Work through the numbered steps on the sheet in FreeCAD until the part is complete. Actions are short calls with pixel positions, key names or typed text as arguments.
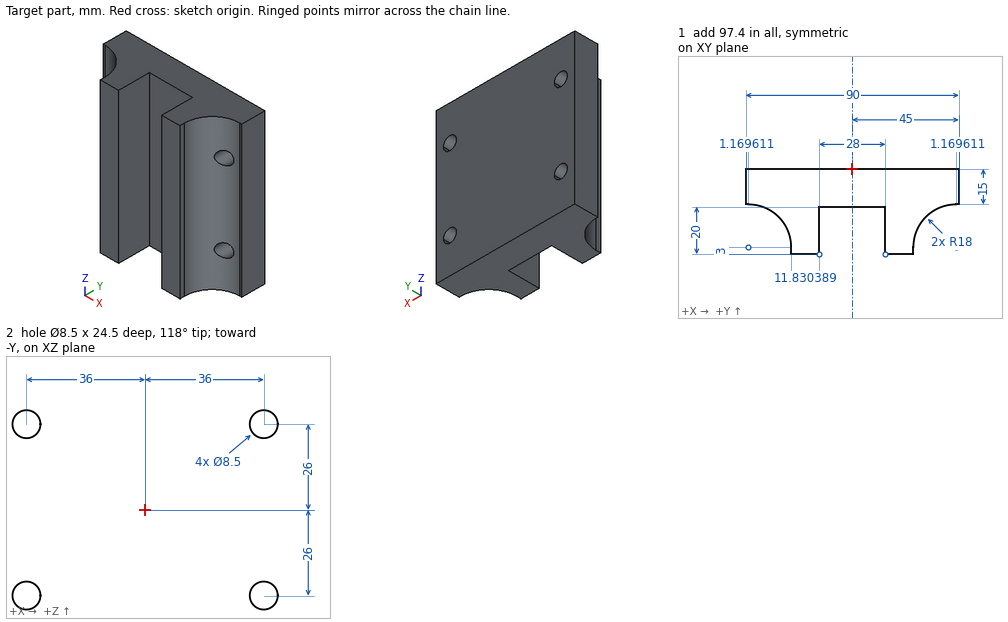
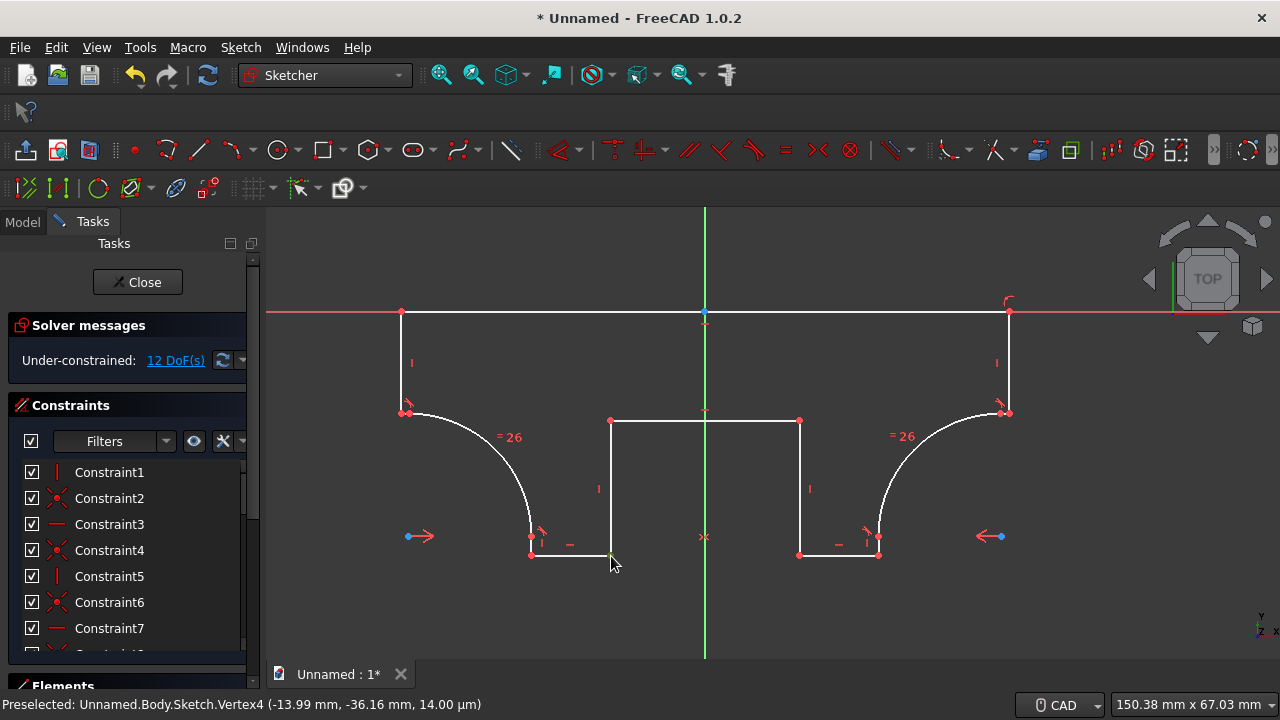
click(800, 556)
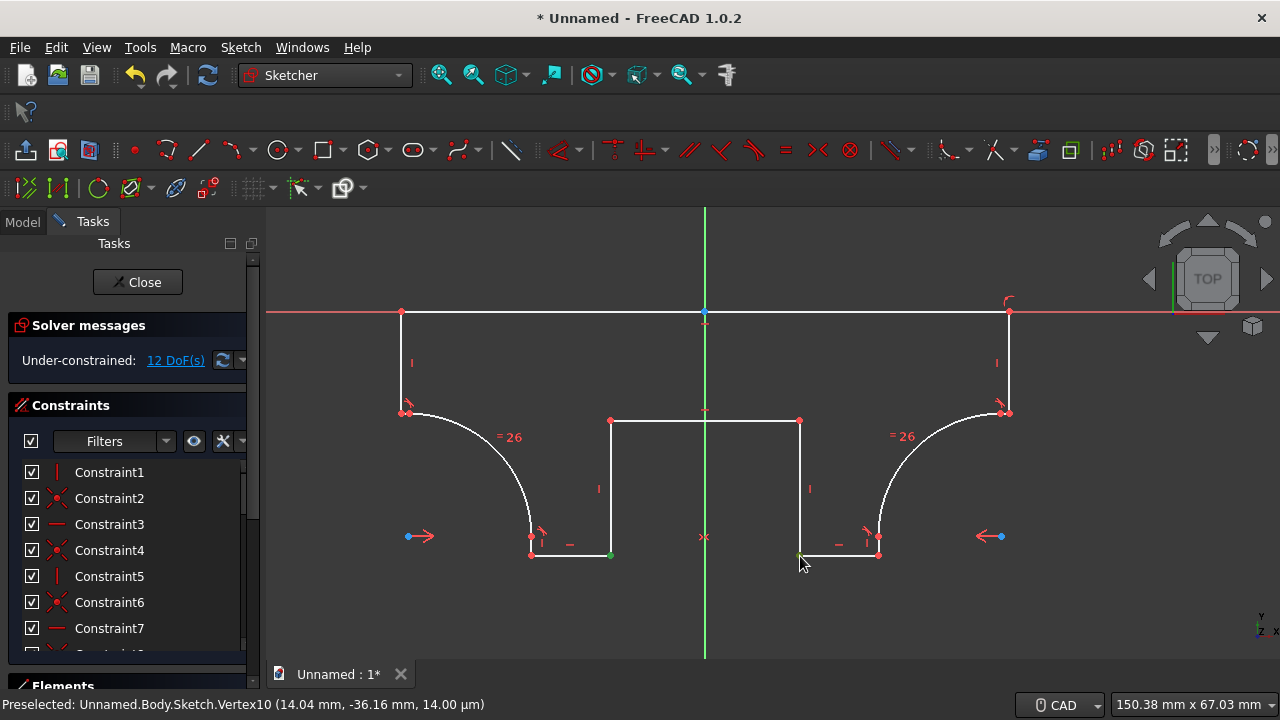
click(705, 603)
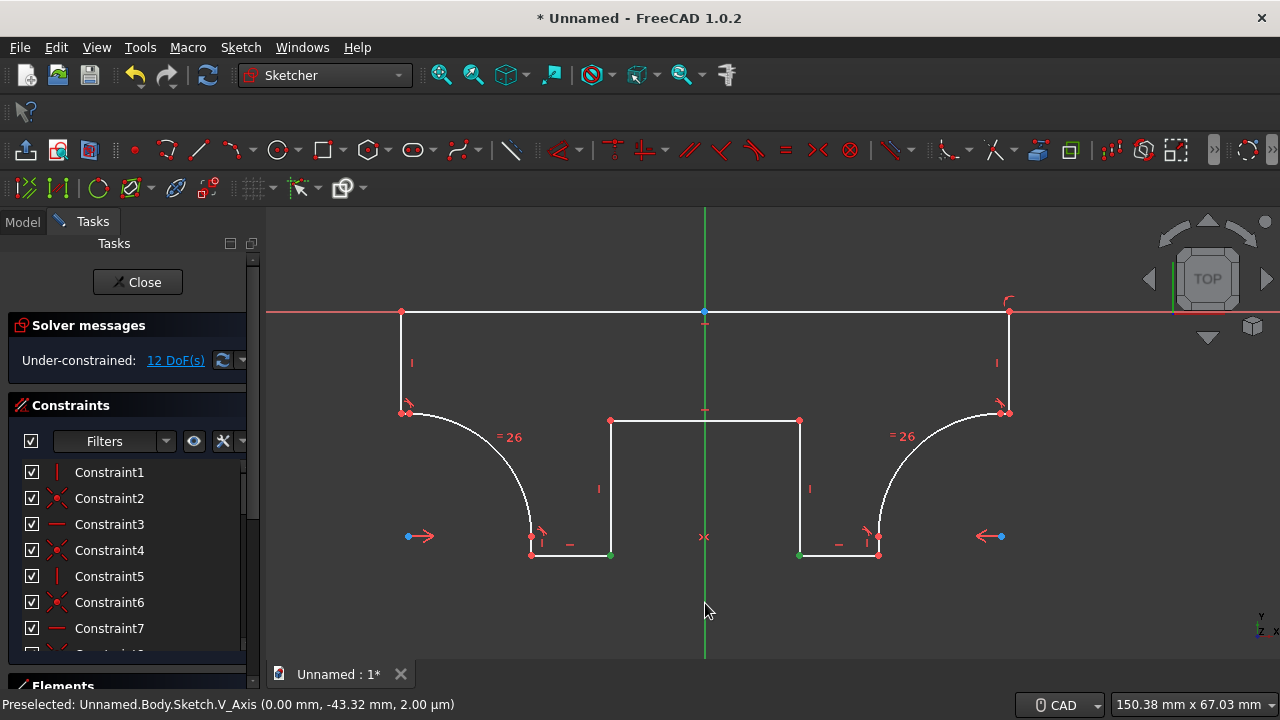
click(818, 150)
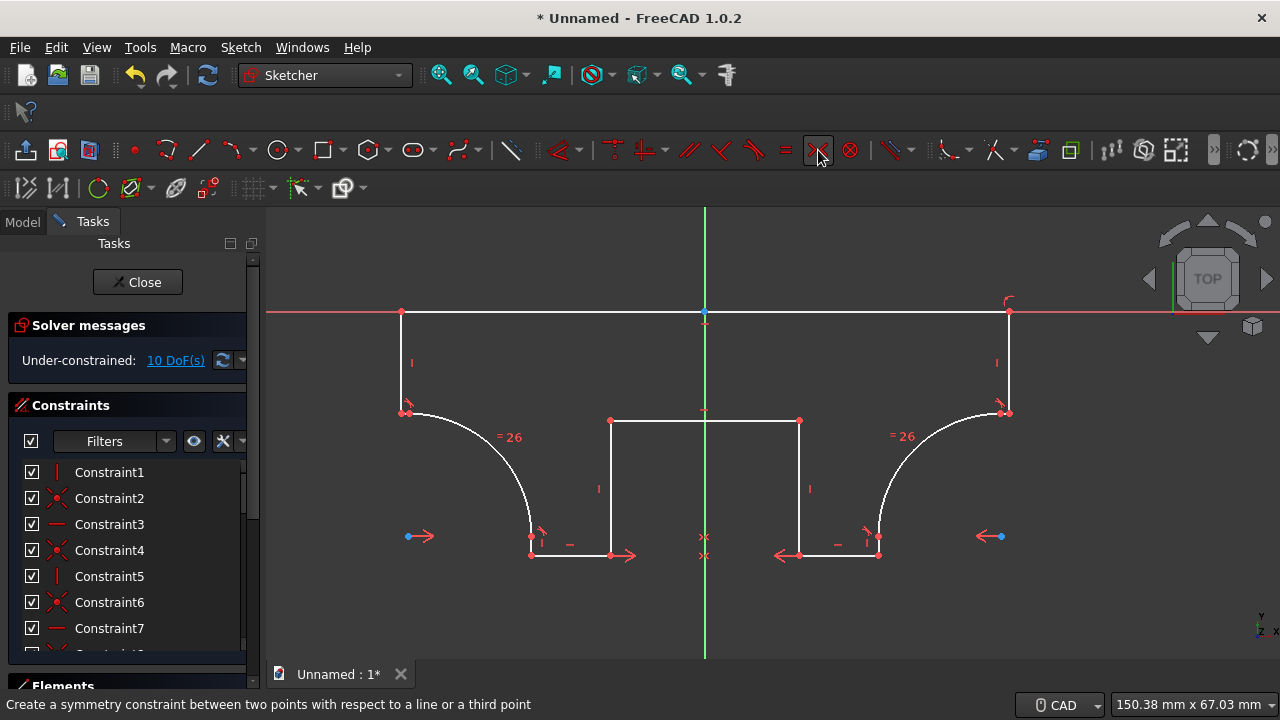
click(945, 427)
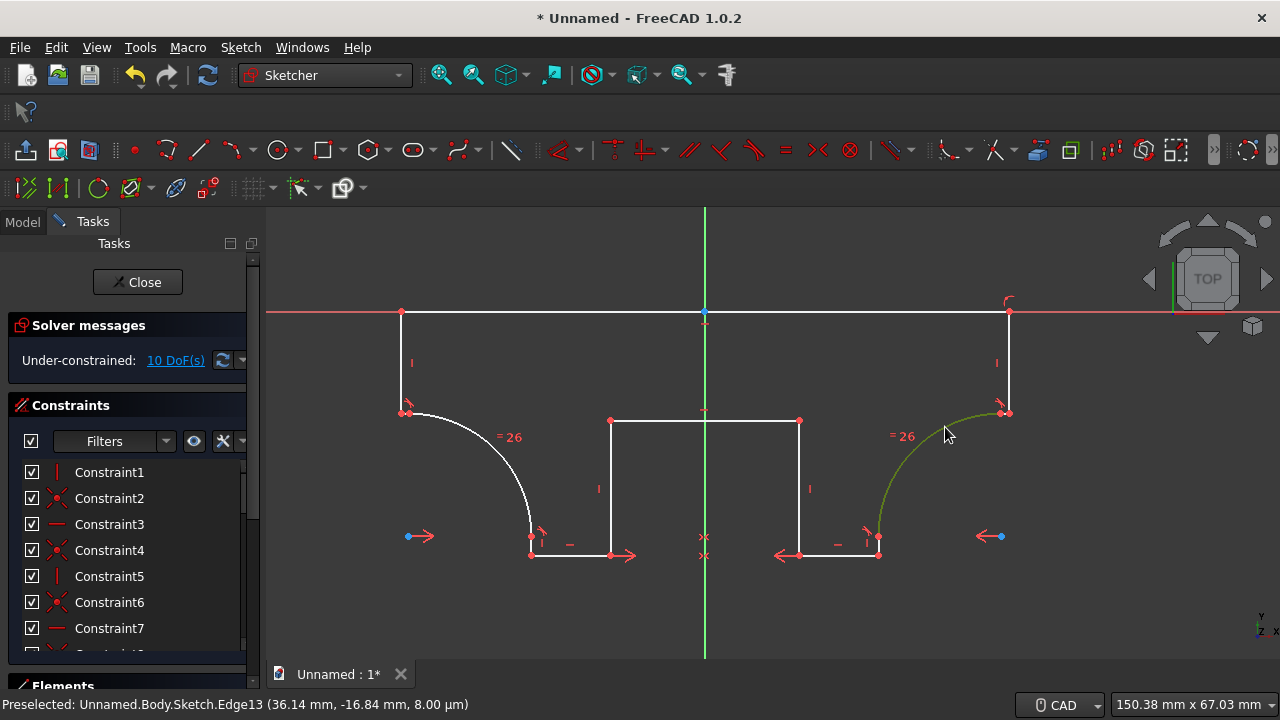
click(582, 150)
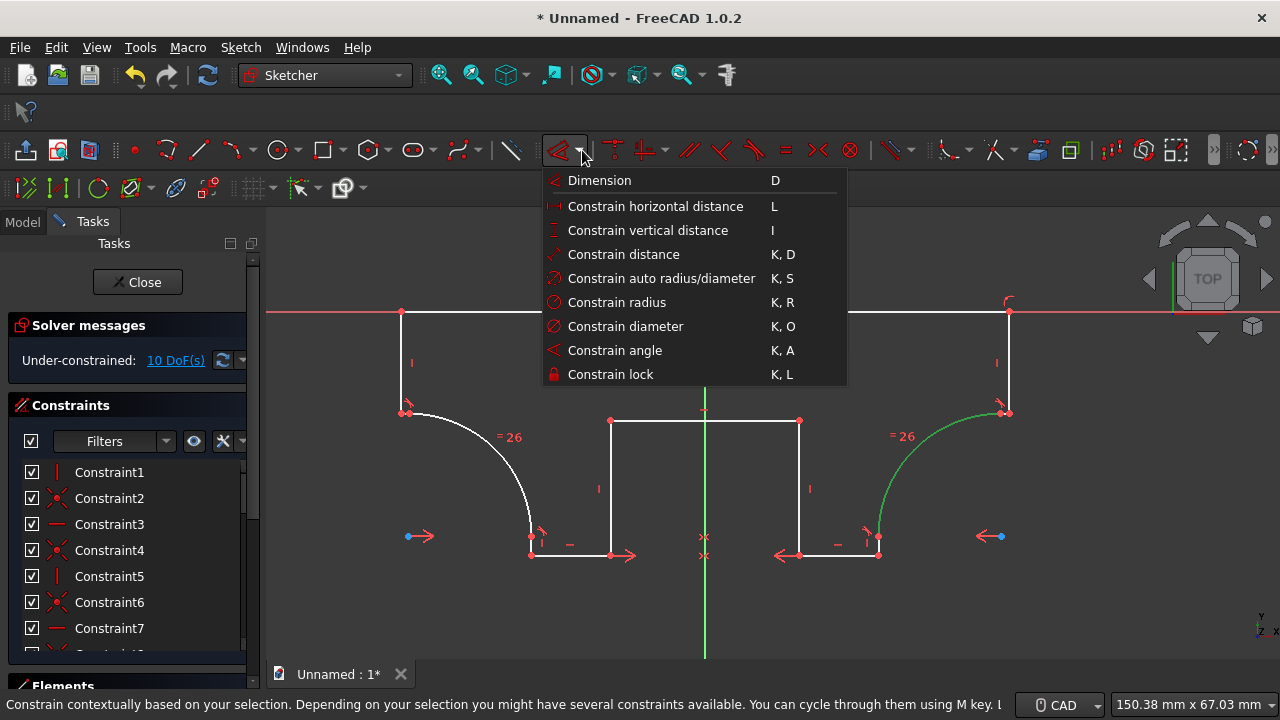
click(695, 302)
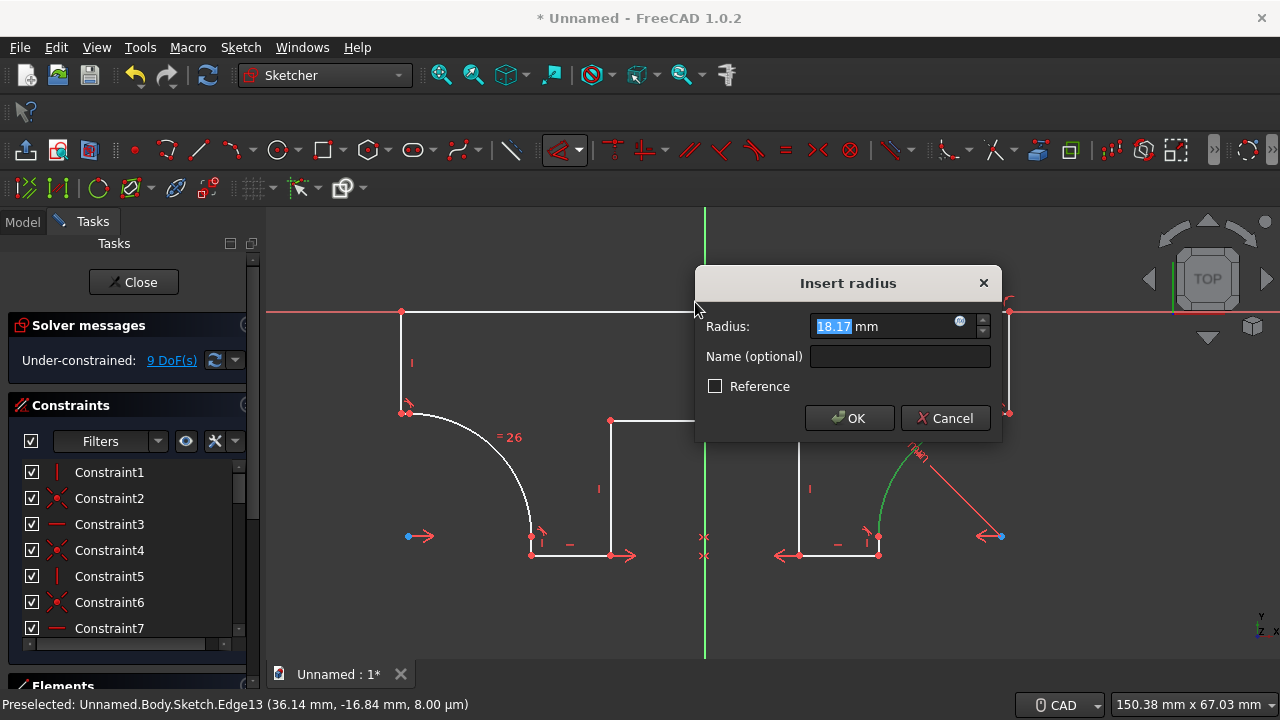
text(18)
key(Return)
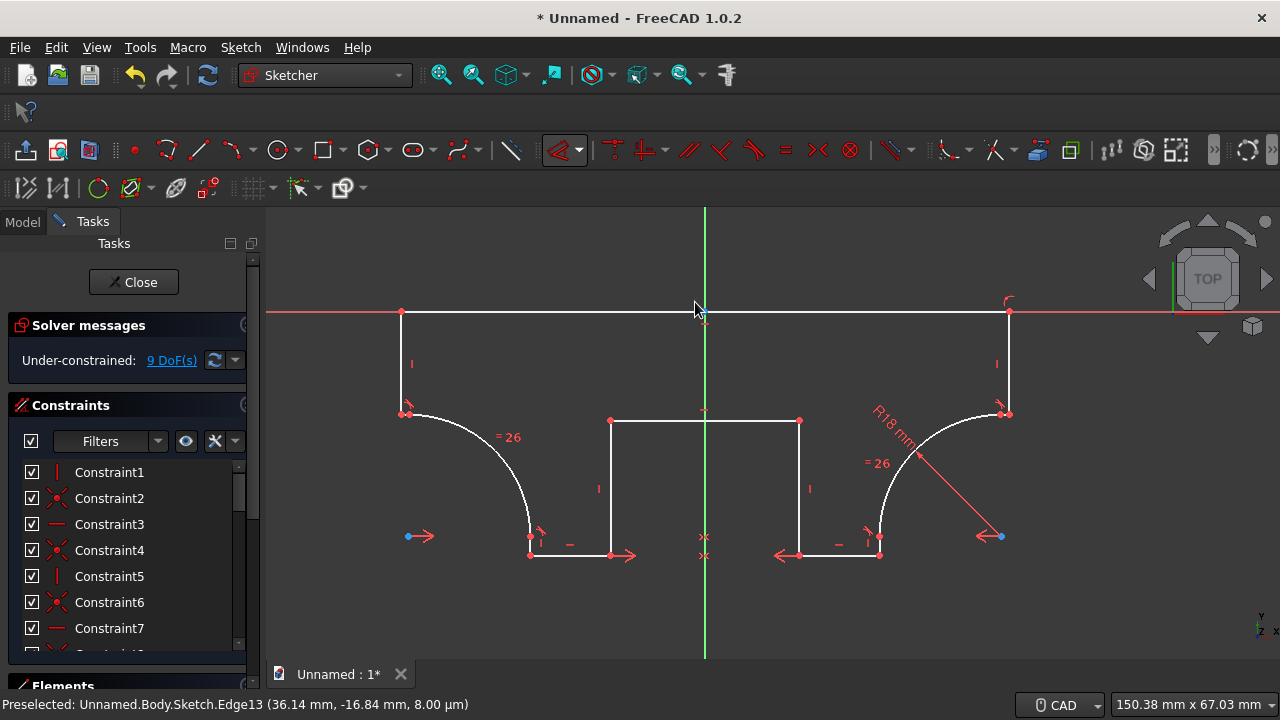
scroll(530, 546, up, 4)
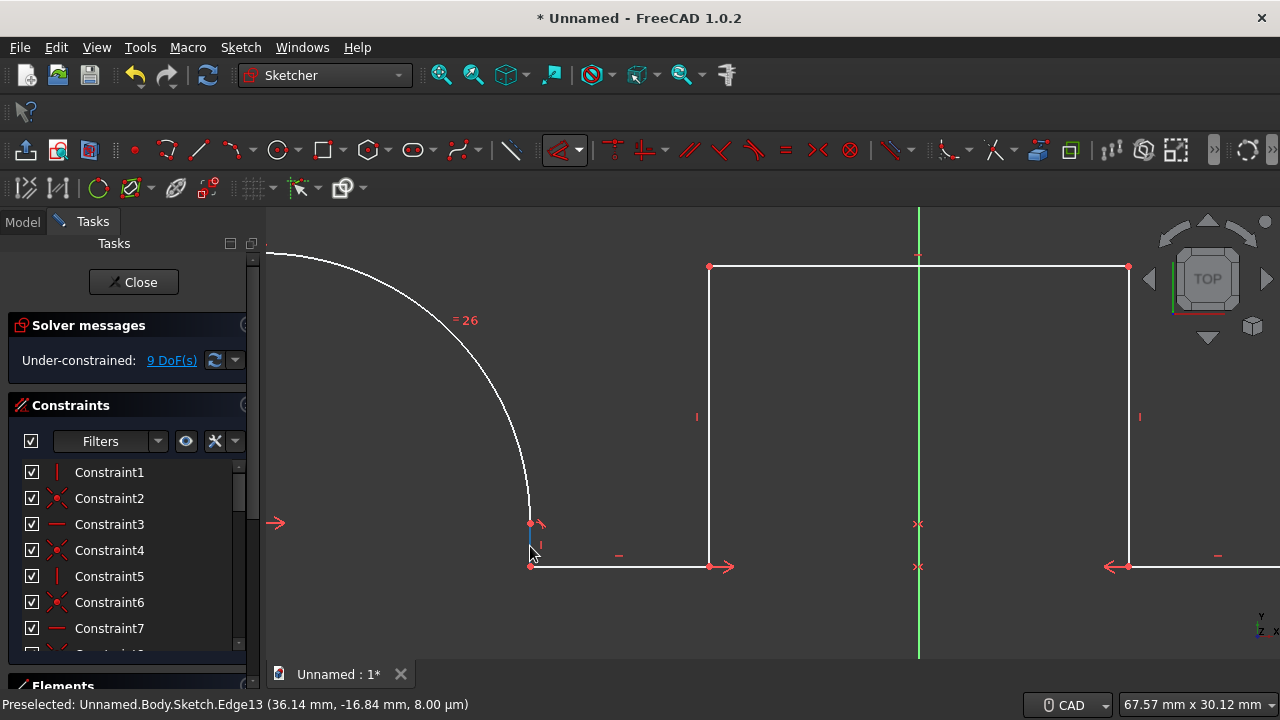
click(530, 545)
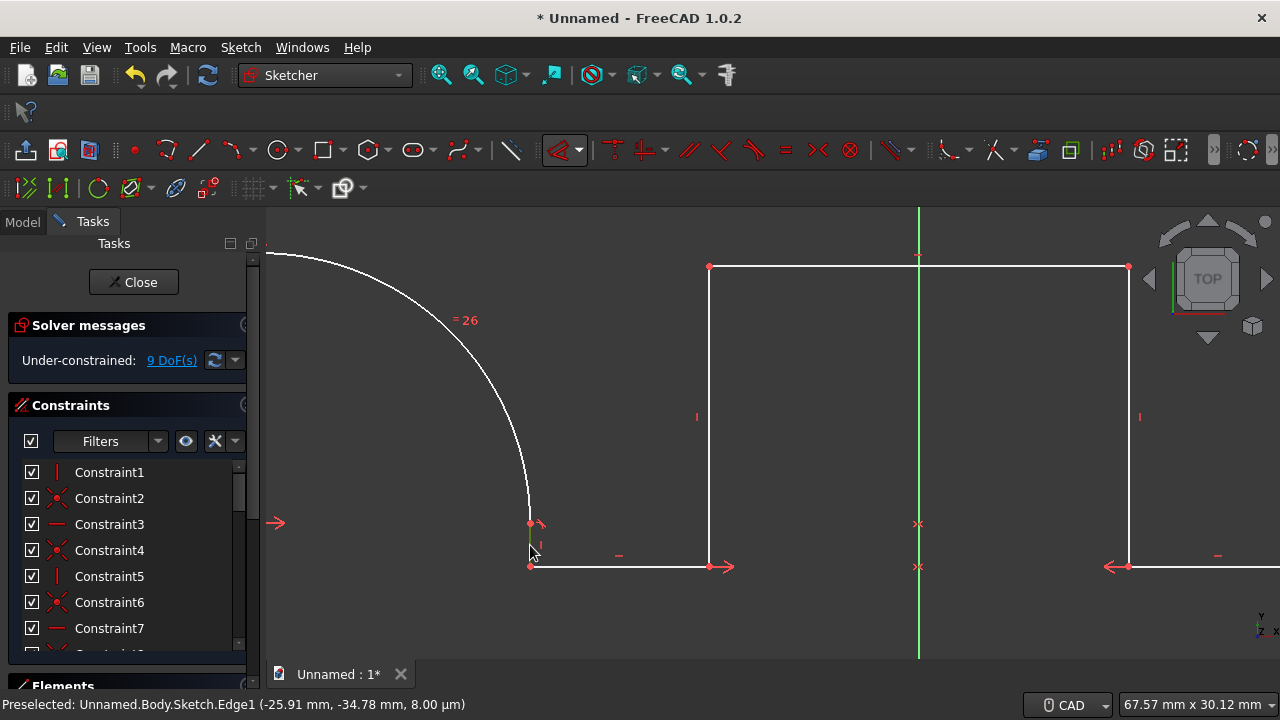
key(i)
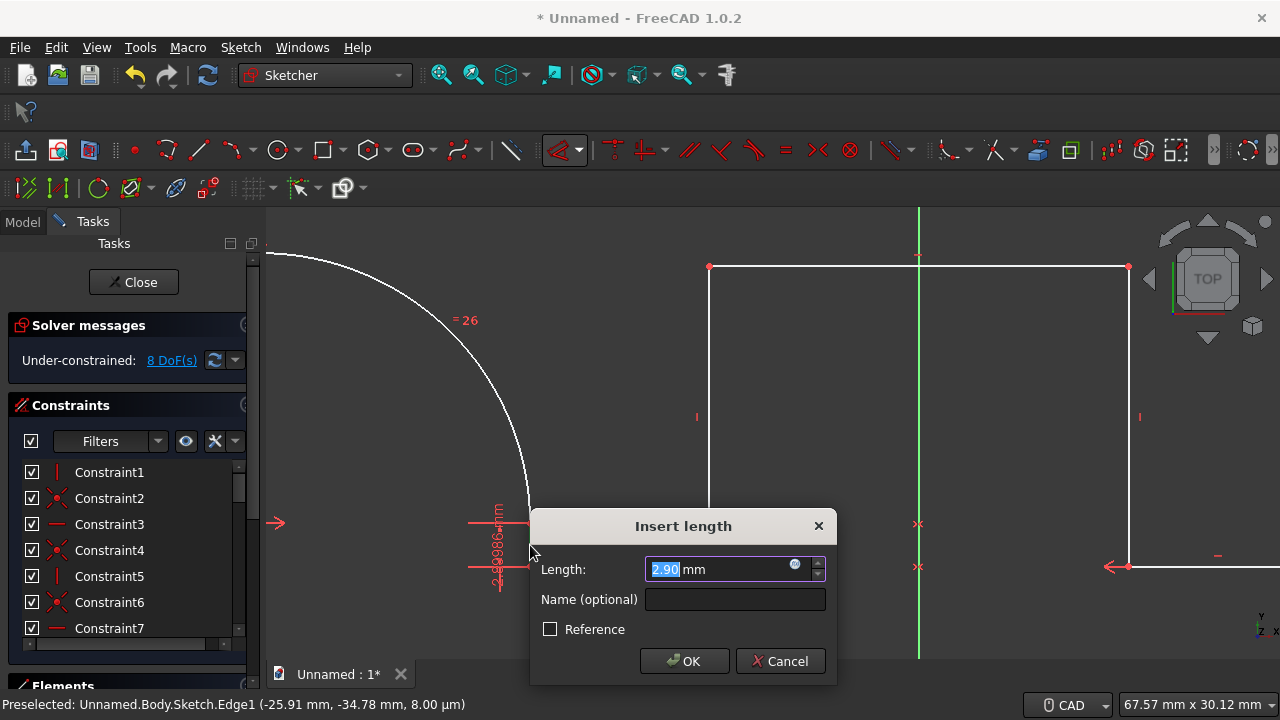
text(3)
key(Return)